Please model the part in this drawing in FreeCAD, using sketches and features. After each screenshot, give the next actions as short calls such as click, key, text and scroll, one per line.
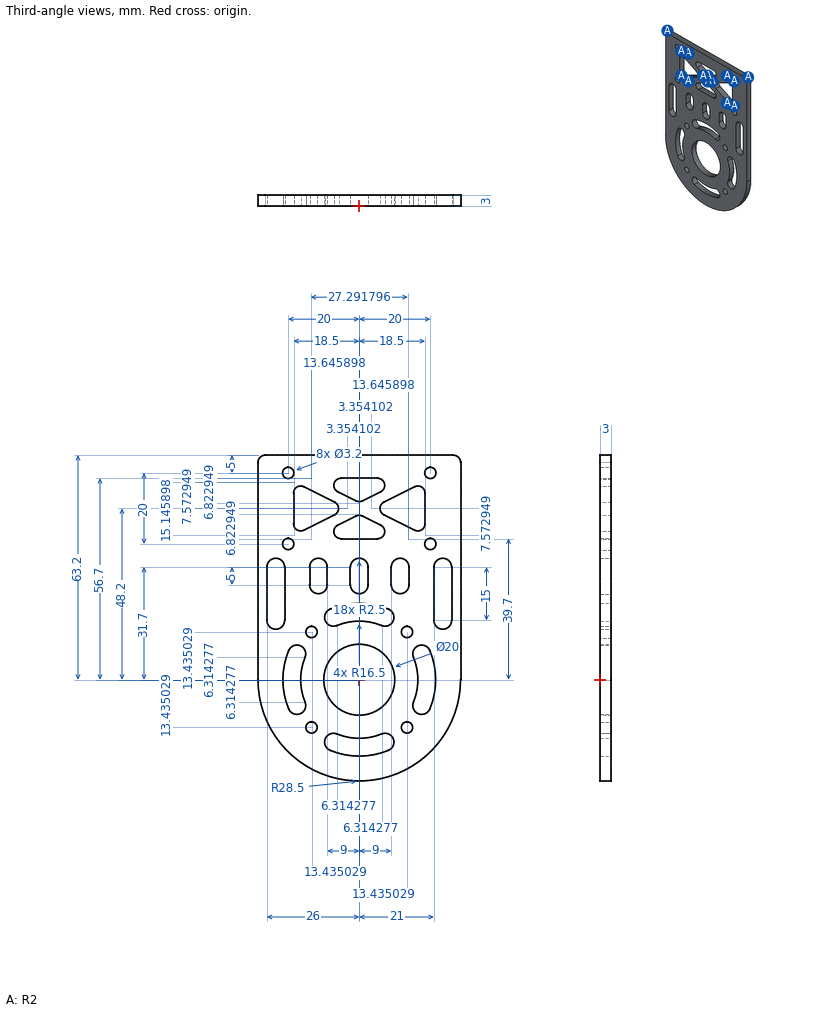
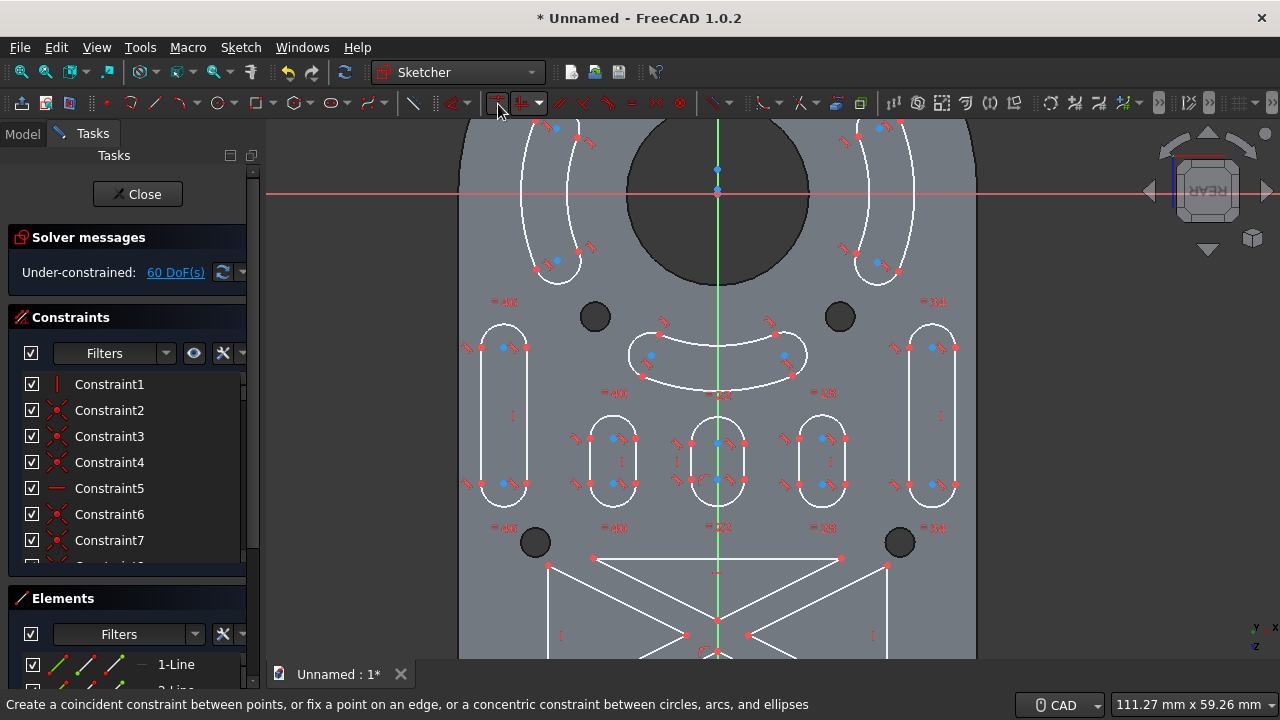
click(694, 344)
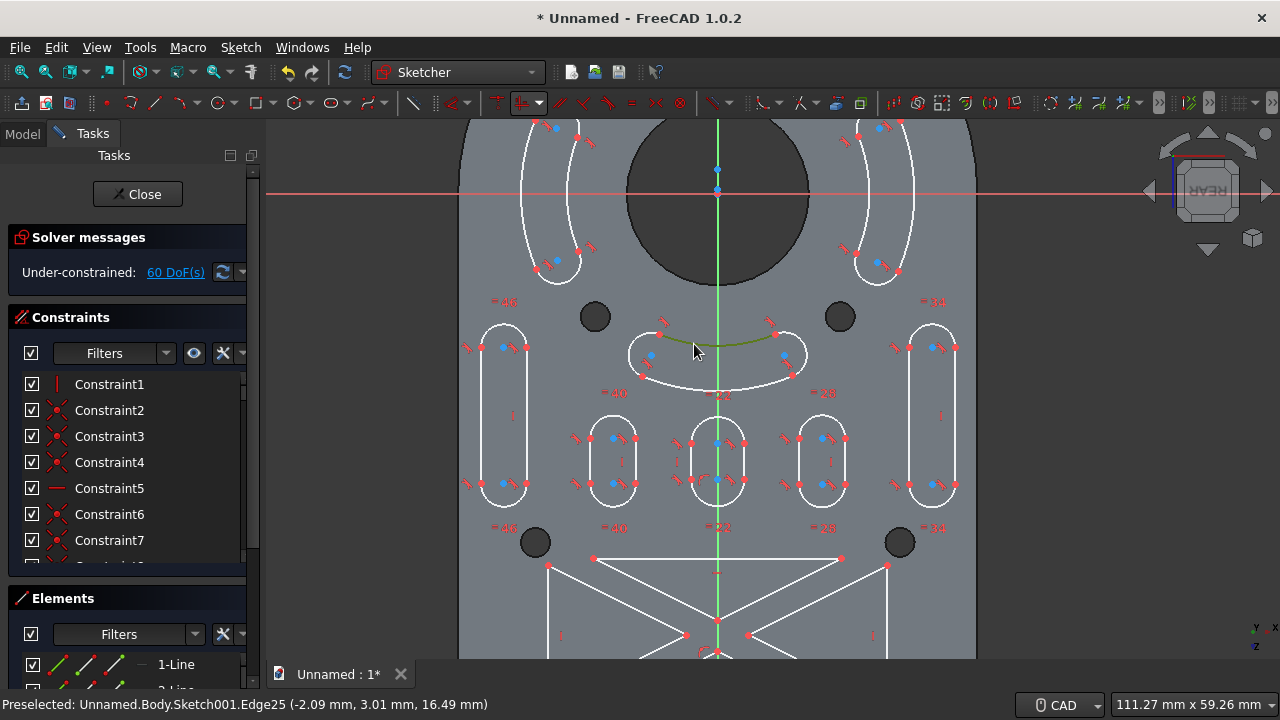
scroll(694, 417, down, 4)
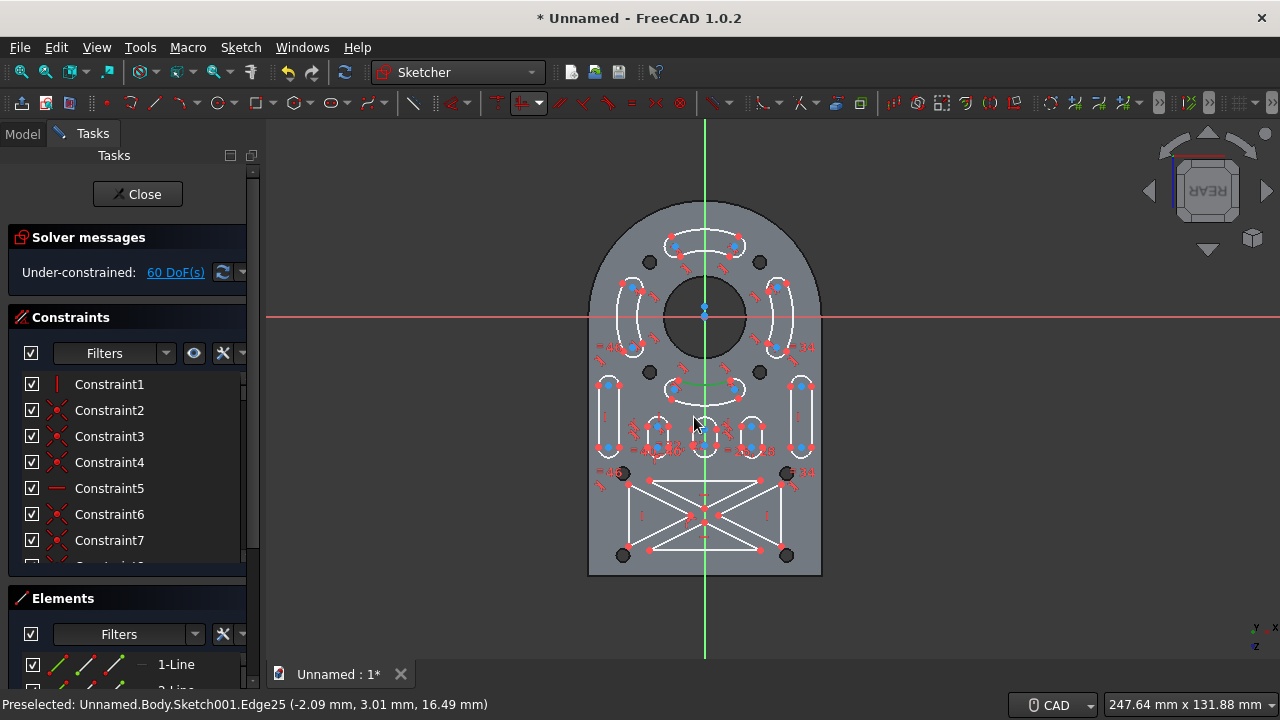
scroll(715, 251, up, 2)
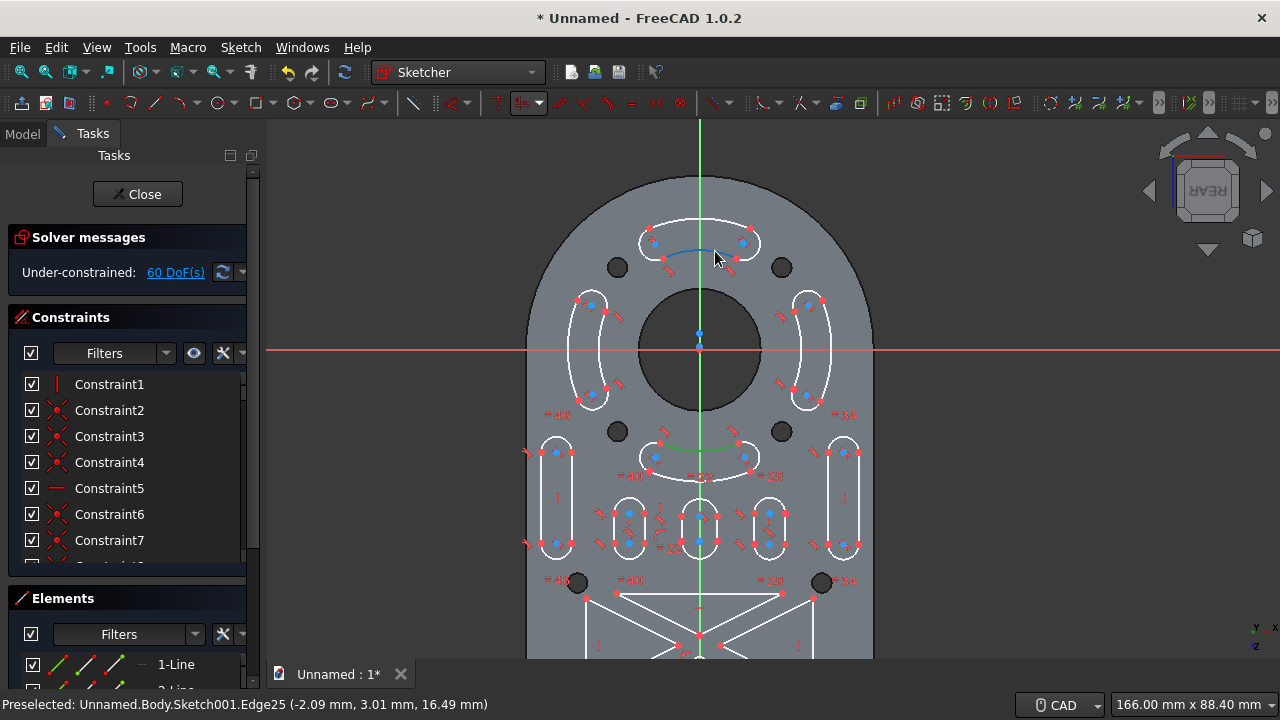
click(715, 252)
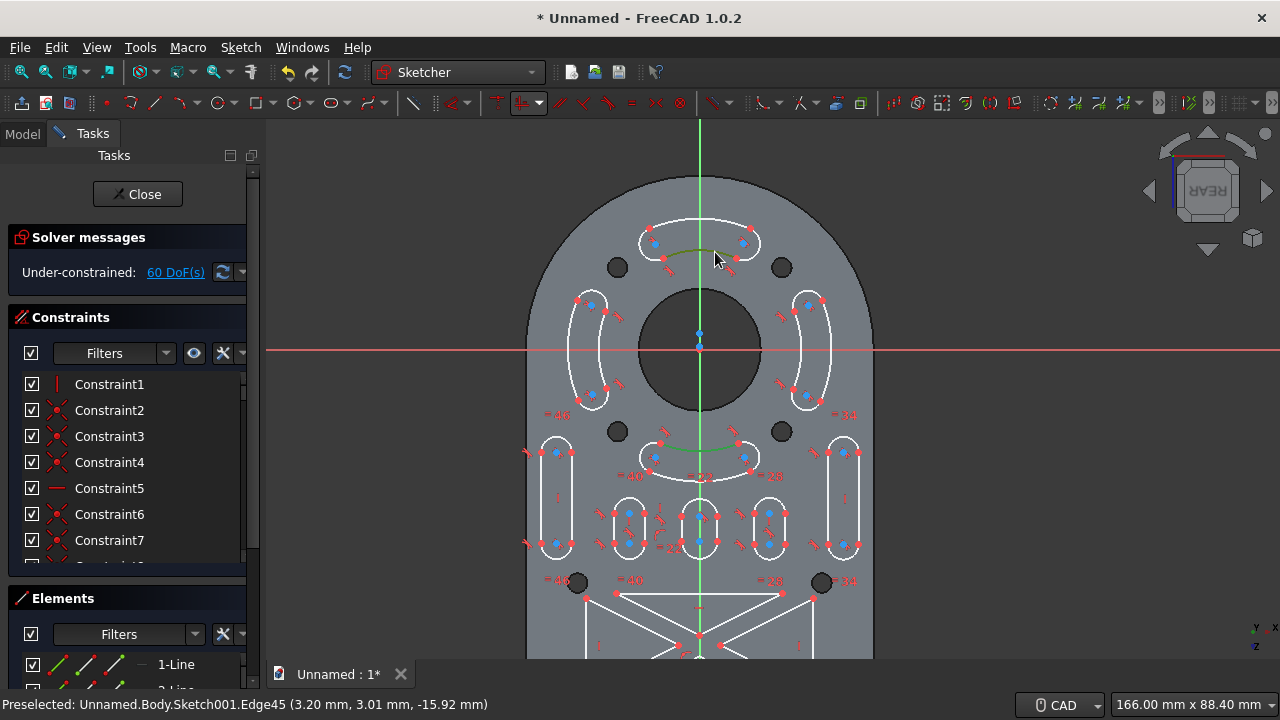
click(498, 104)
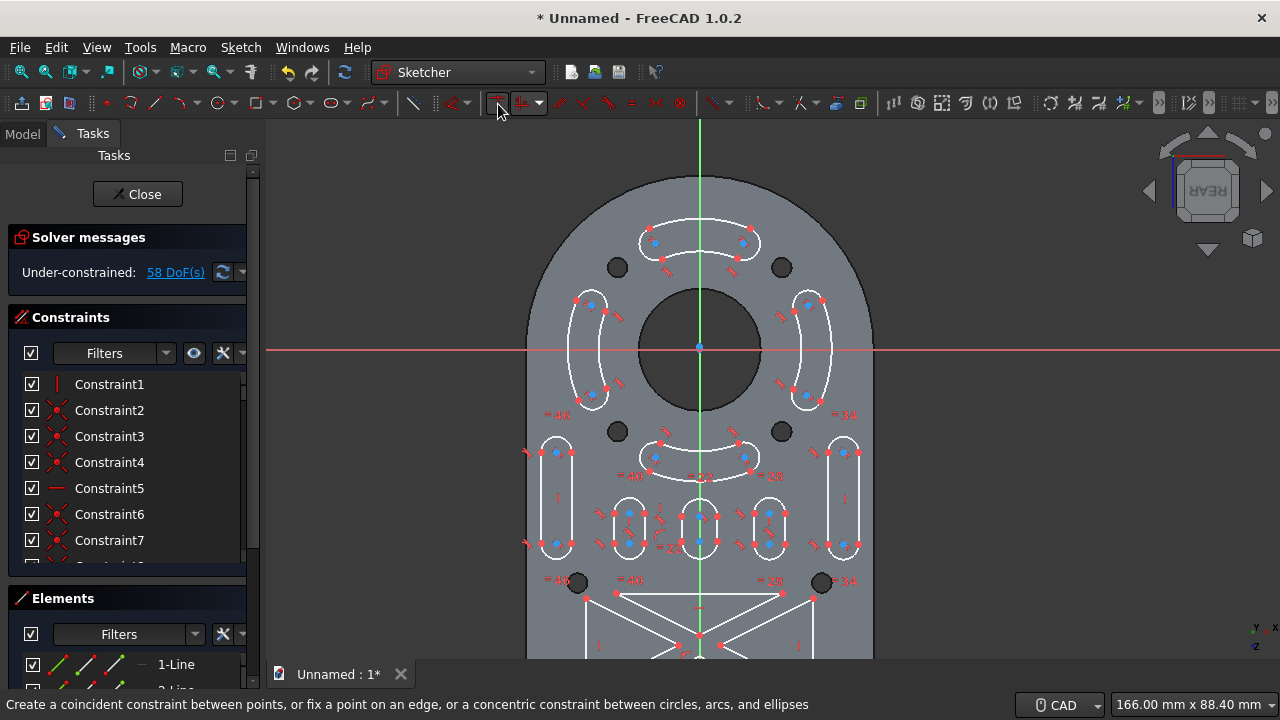
click(684, 450)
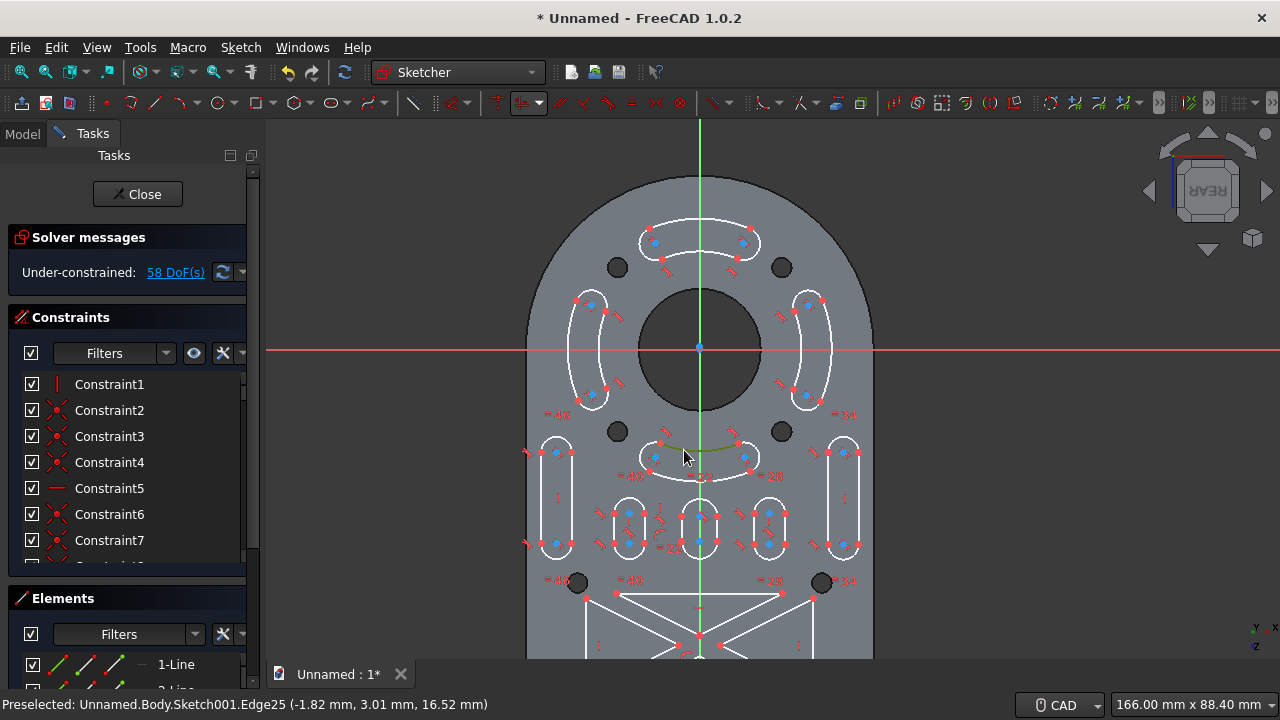
click(720, 220)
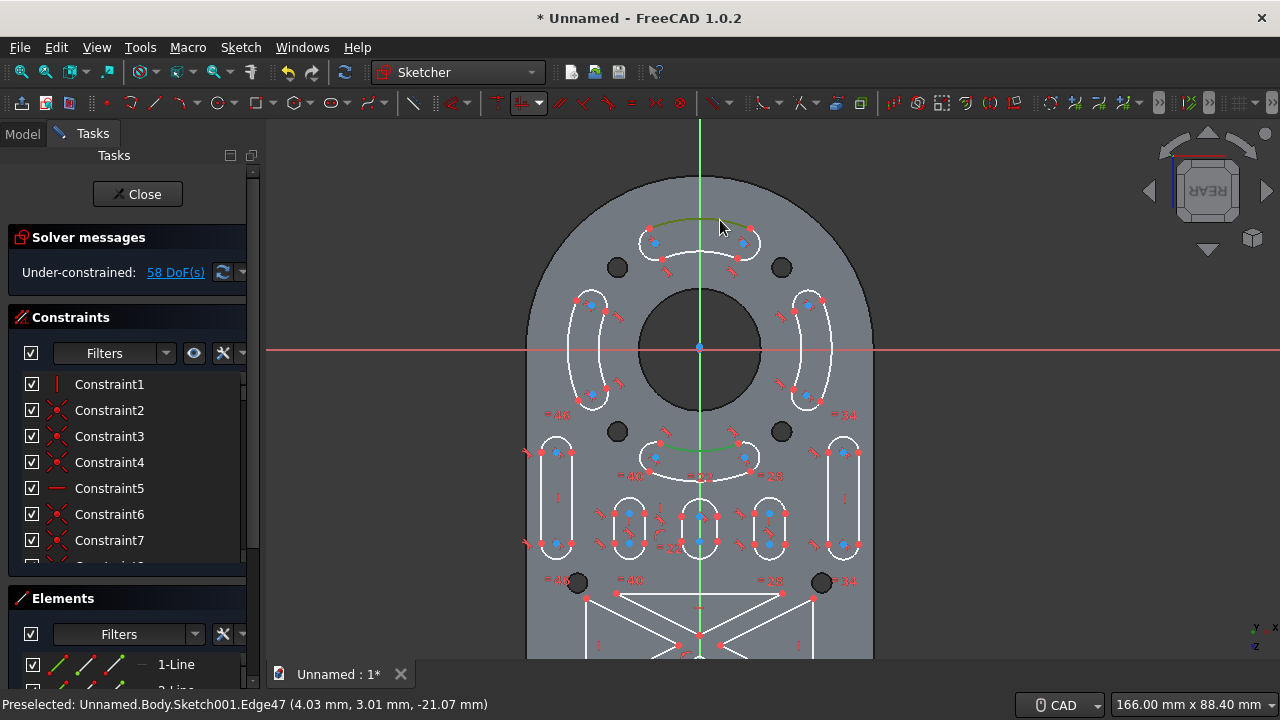
click(498, 104)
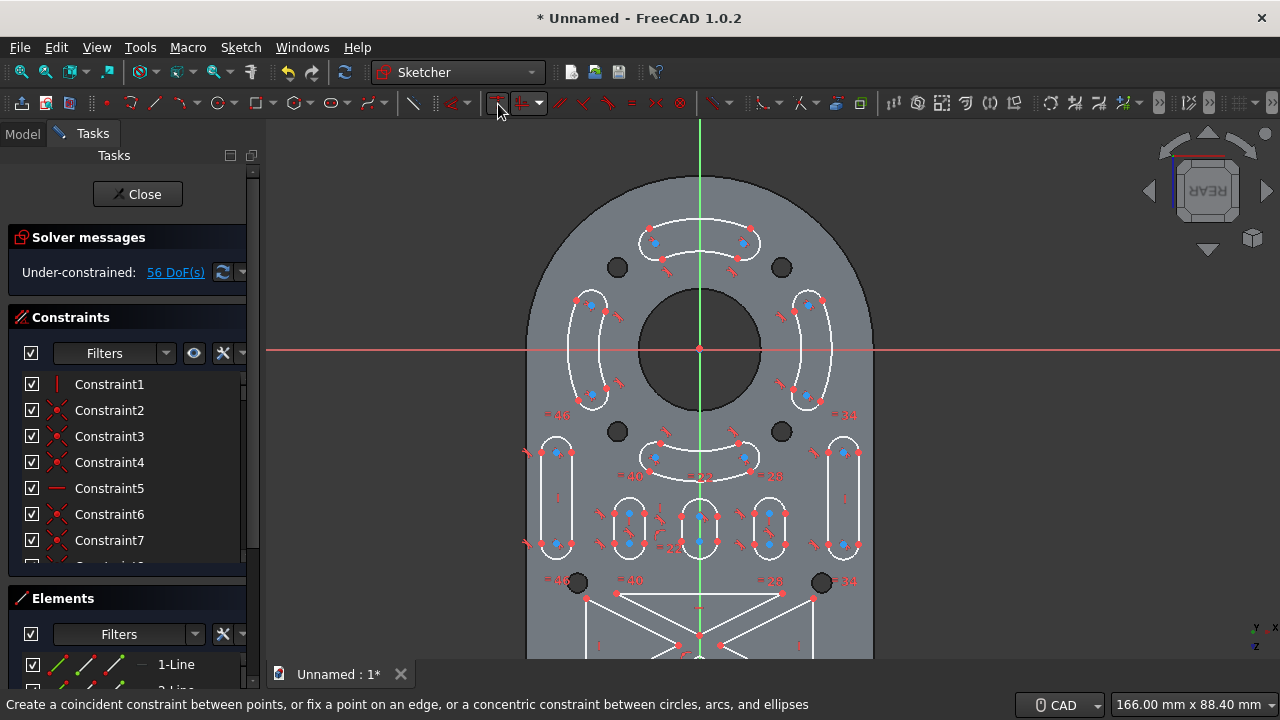
scroll(700, 349, up, 5)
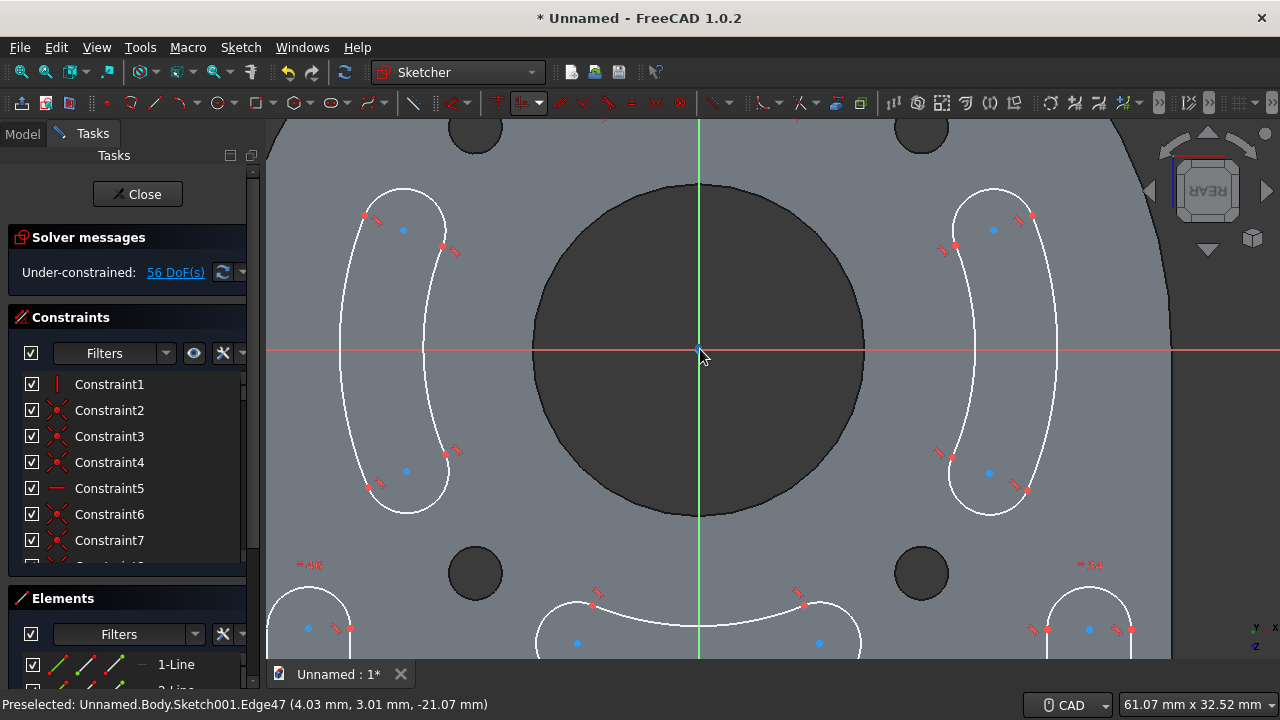
drag(689, 337, 709, 360)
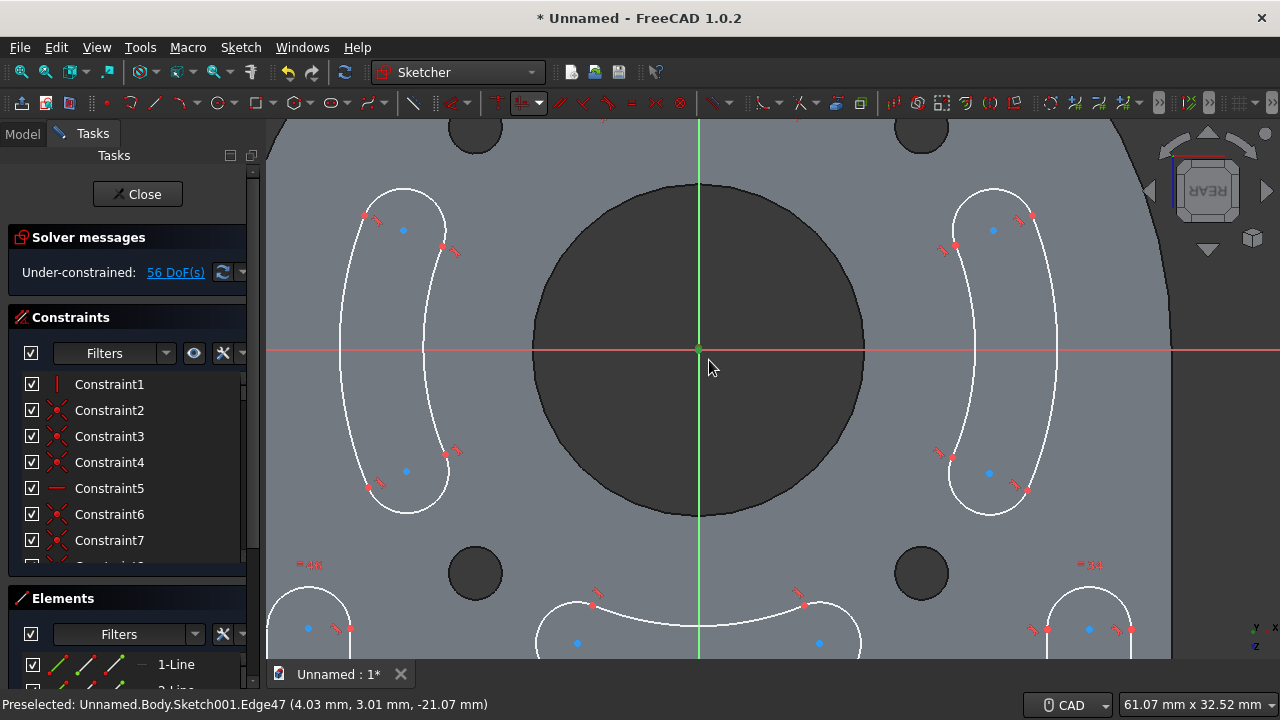
click(498, 104)